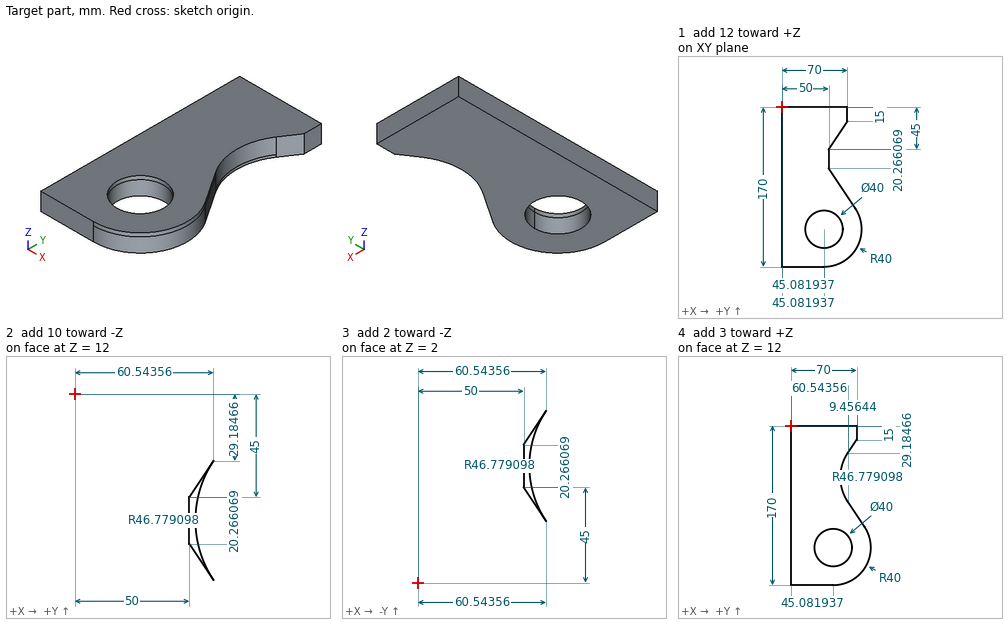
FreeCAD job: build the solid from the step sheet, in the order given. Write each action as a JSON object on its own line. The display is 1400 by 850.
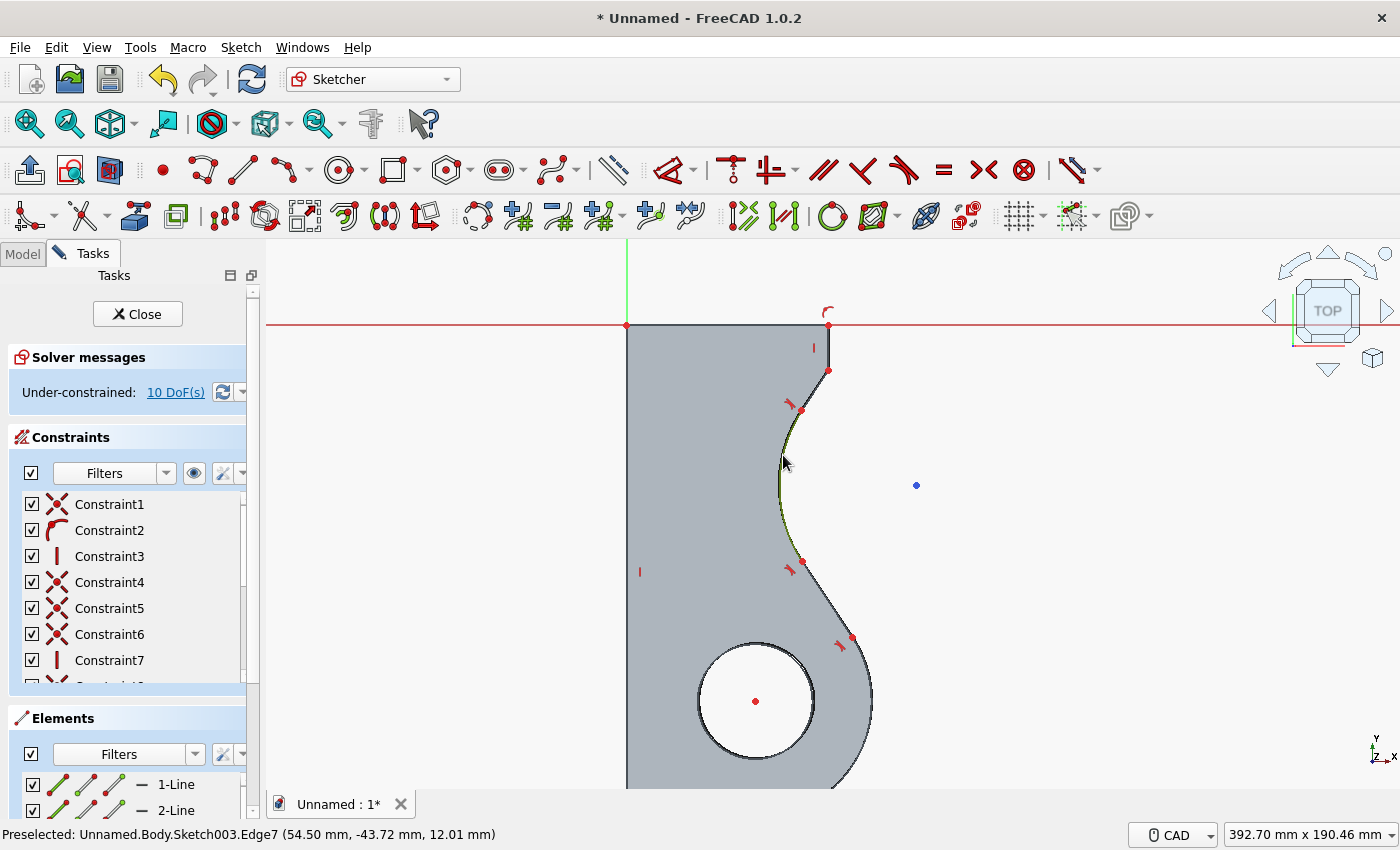
{"action": "left_click", "coordinate": [696, 170]}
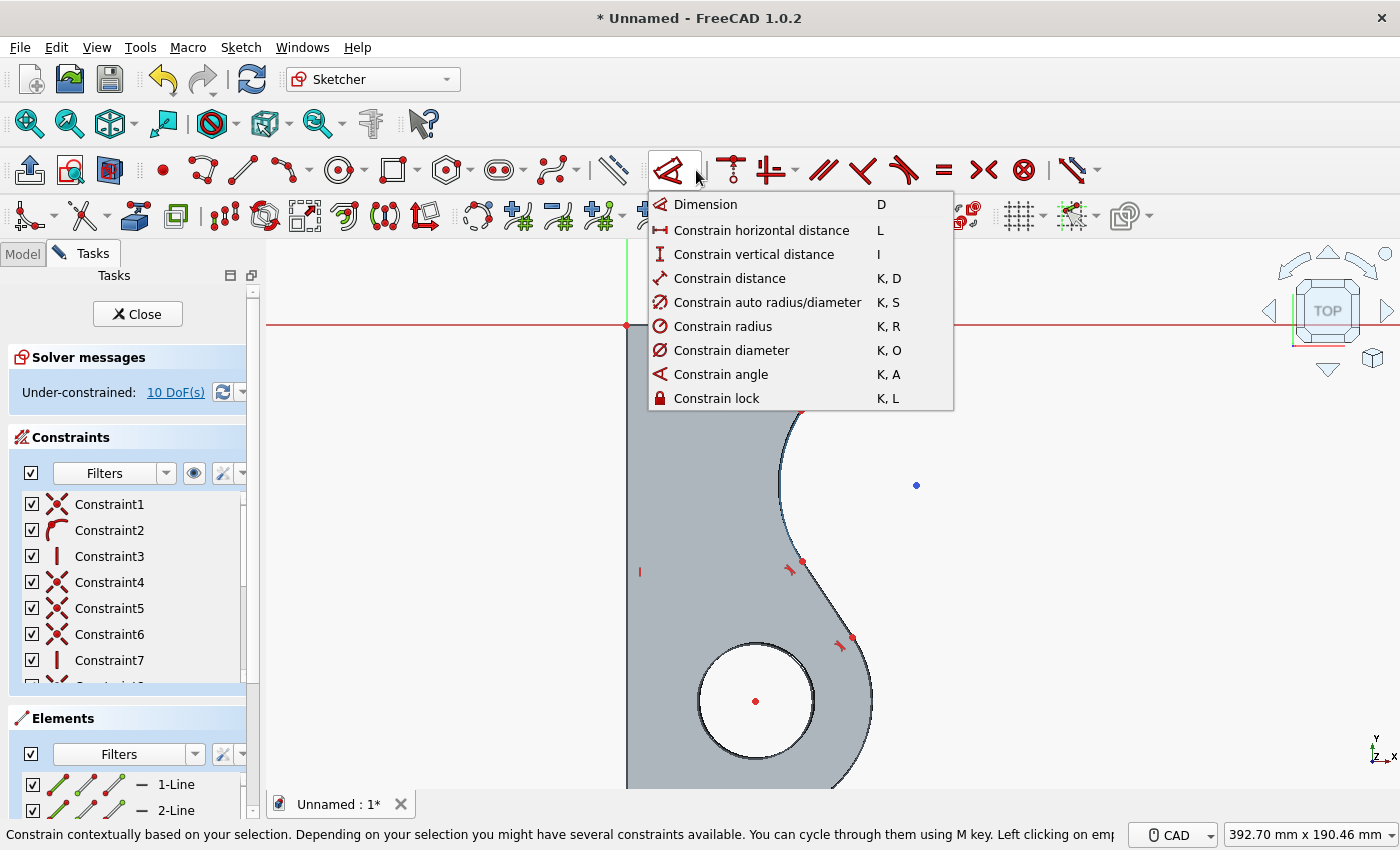
{"action": "left_click", "coordinate": [801, 326]}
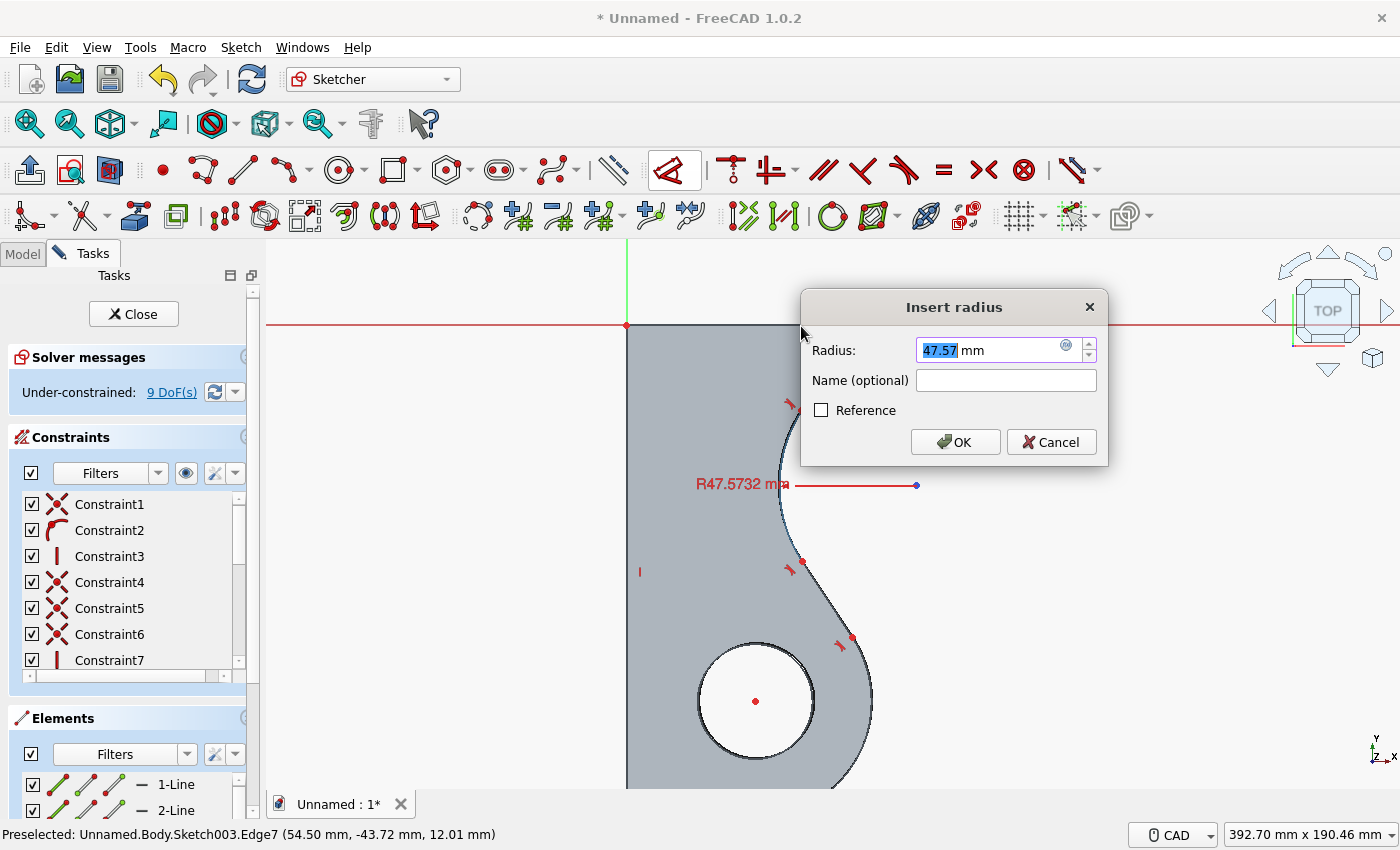
{"action": "type", "text": "46.779098"}
{"action": "key", "text": "Return"}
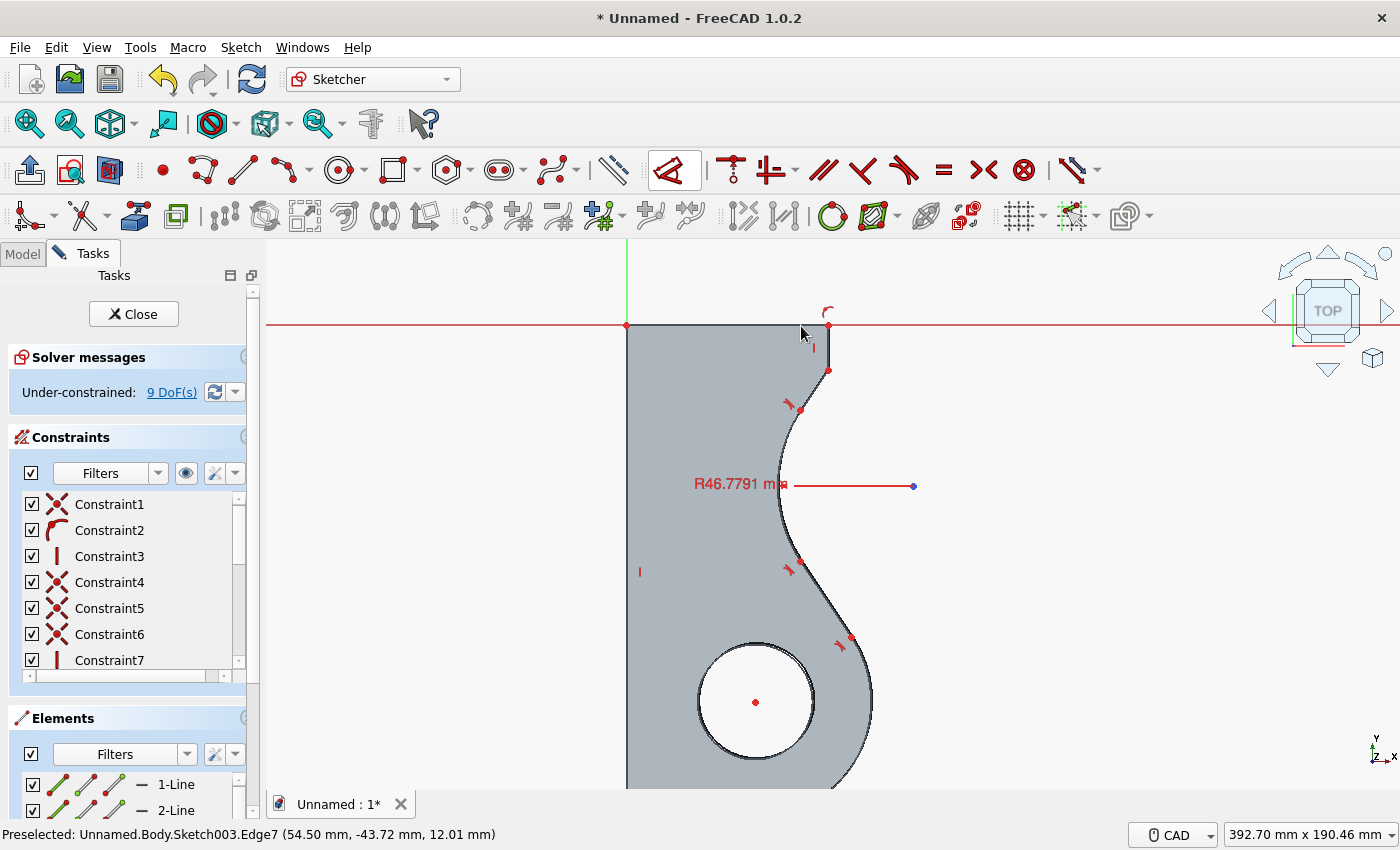
{"action": "left_click", "coordinate": [871, 708]}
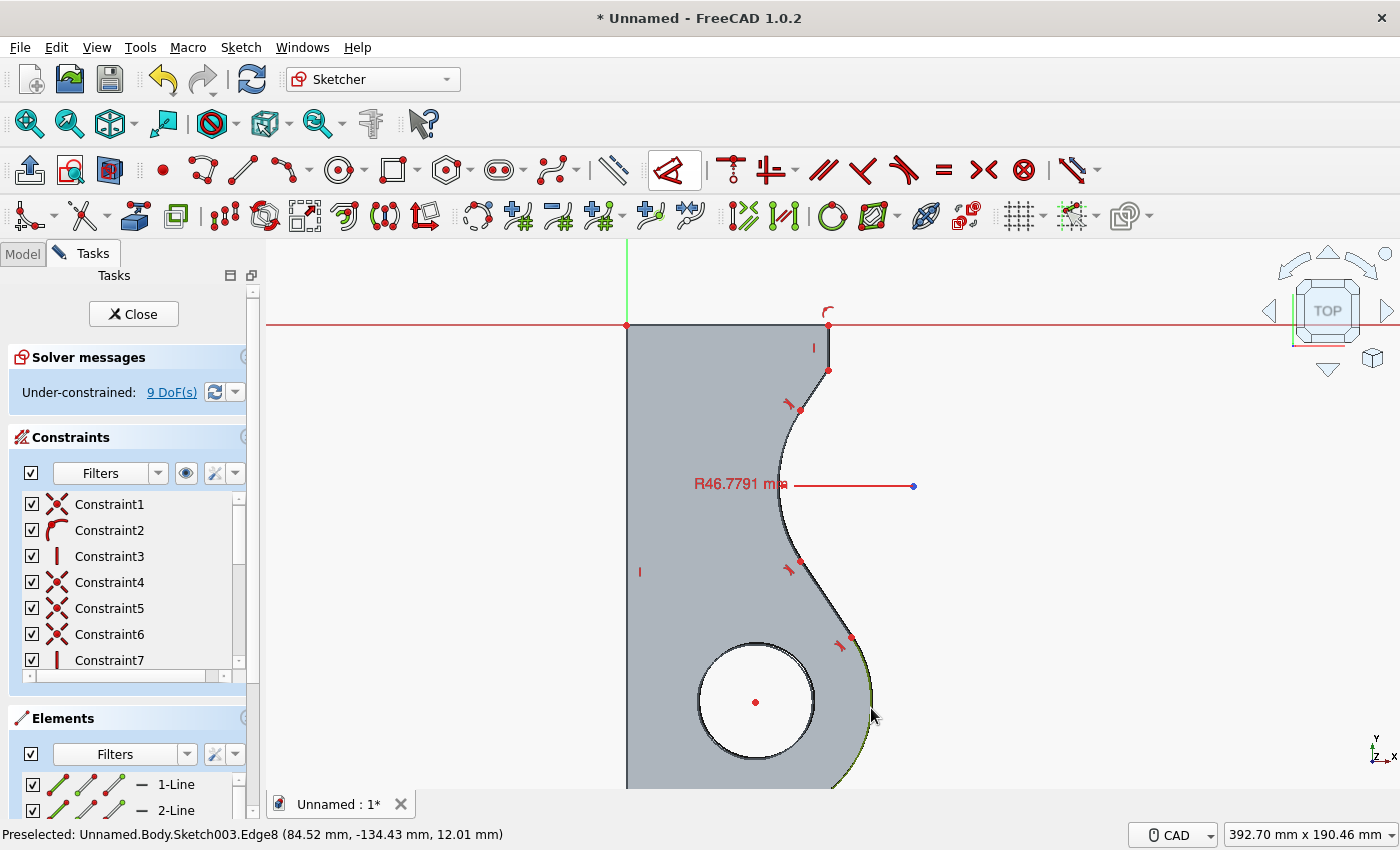
{"action": "key", "text": "k r"}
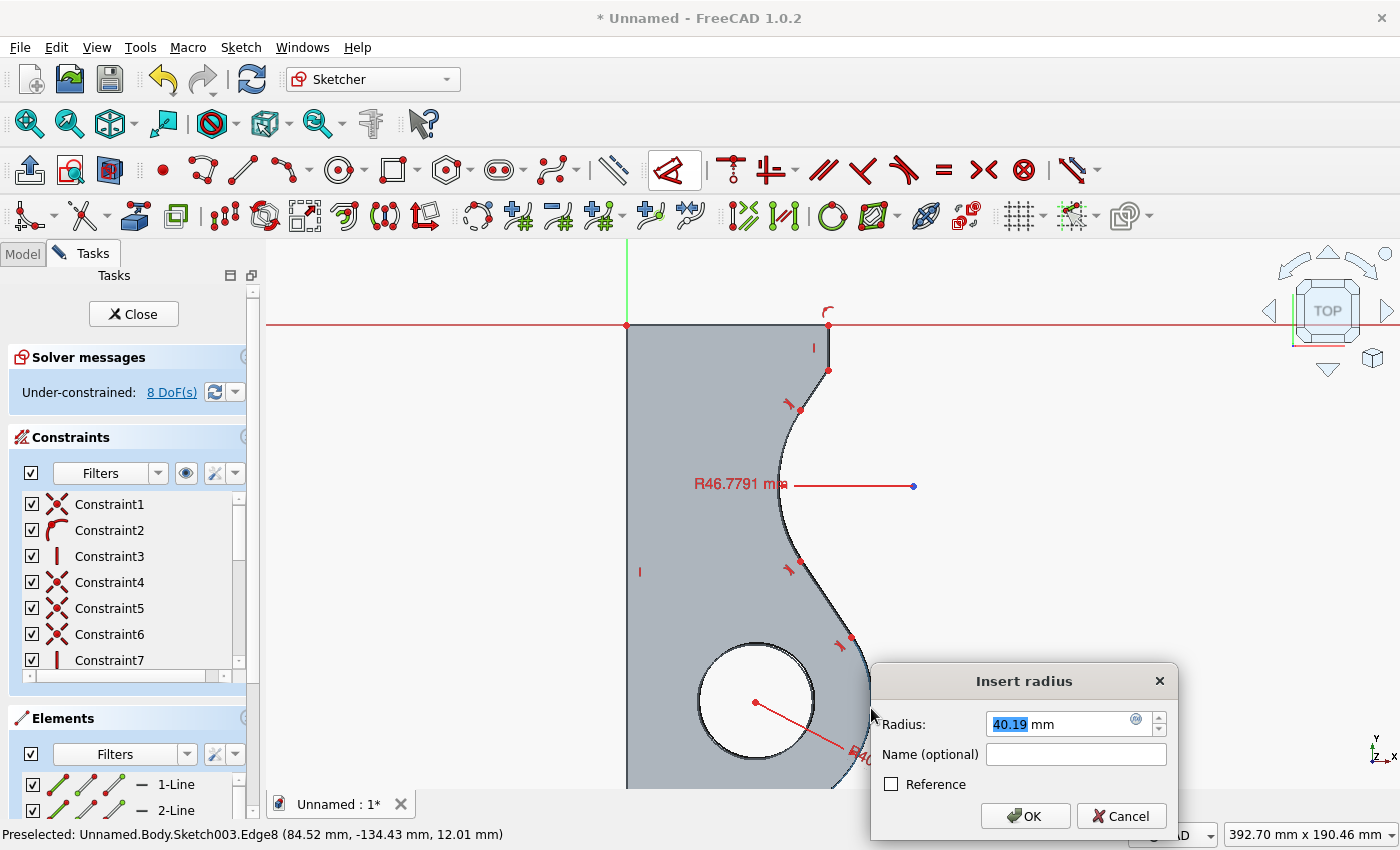
{"action": "type", "text": "40"}
{"action": "key", "text": "Return"}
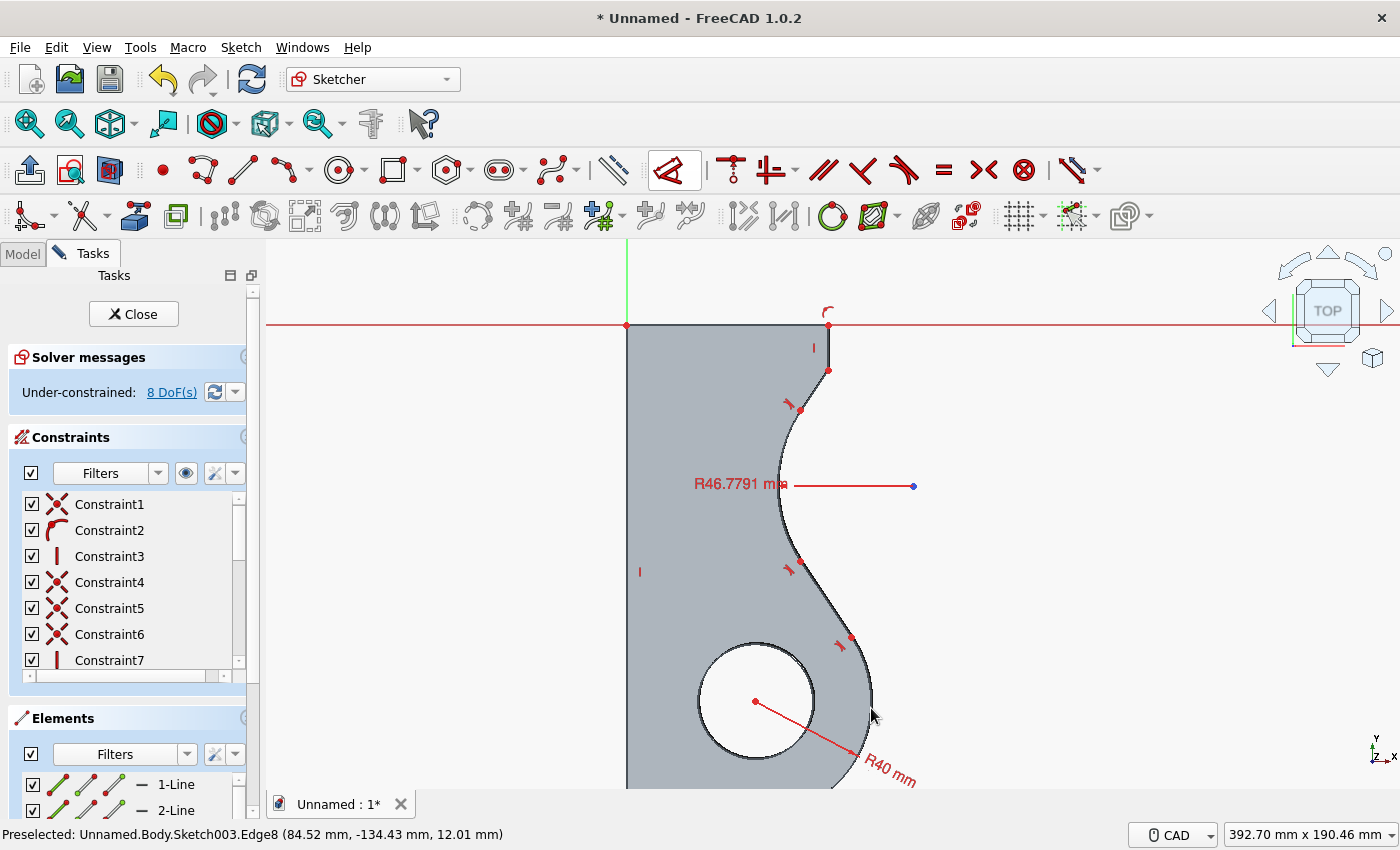
{"action": "left_click", "coordinate": [796, 661]}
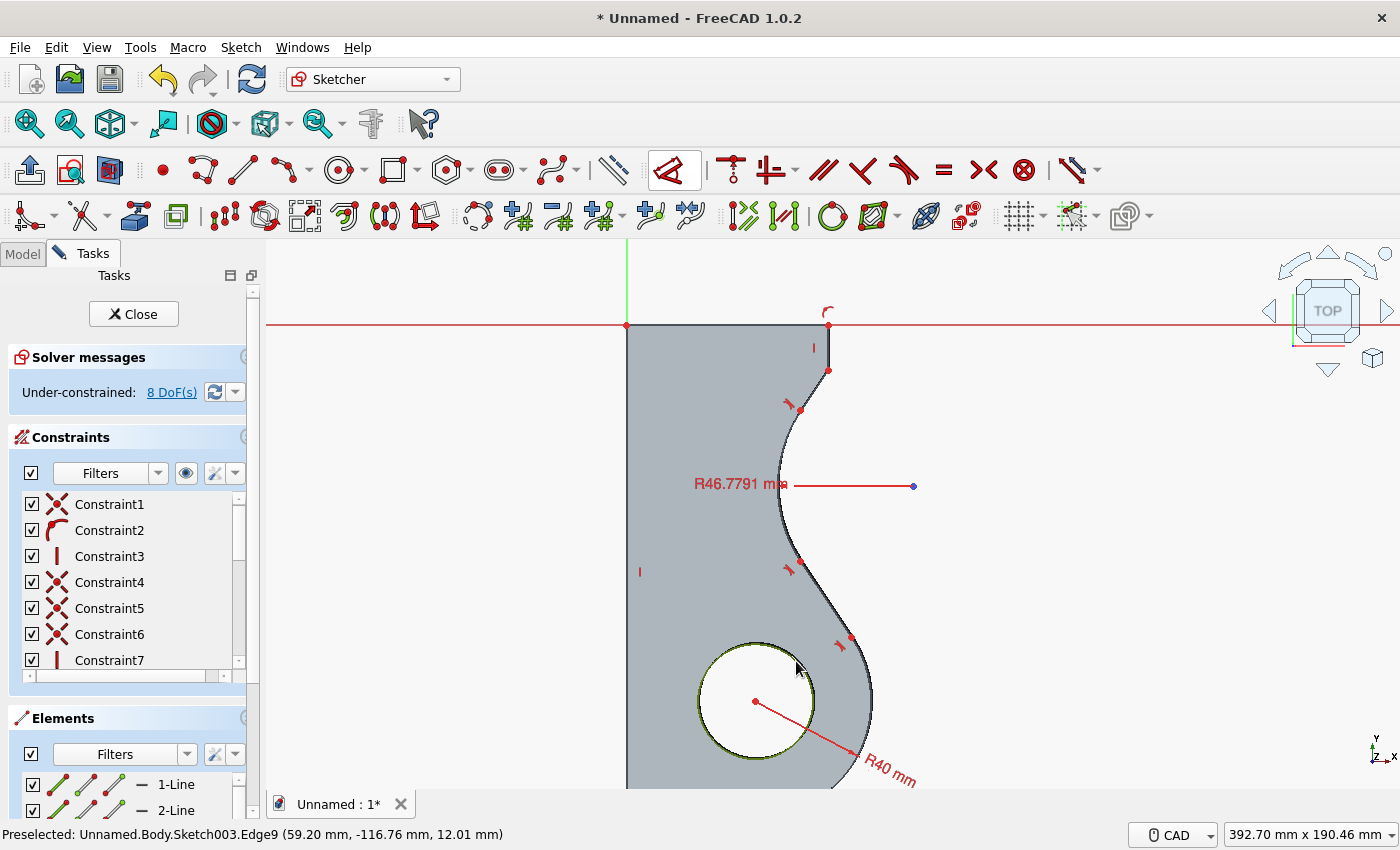
{"action": "key", "text": "k o"}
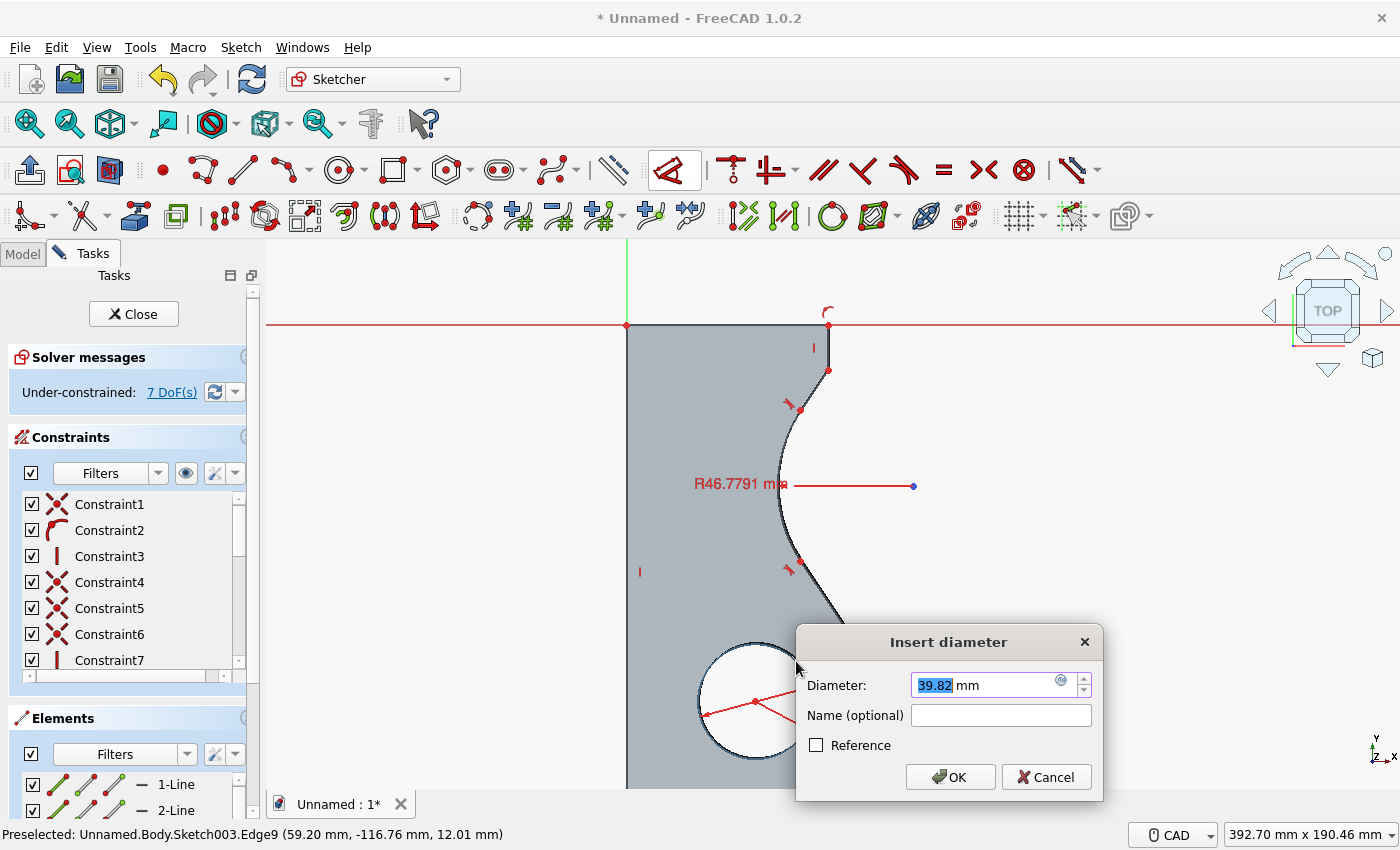
{"action": "type", "text": "40"}
{"action": "key", "text": "Return"}